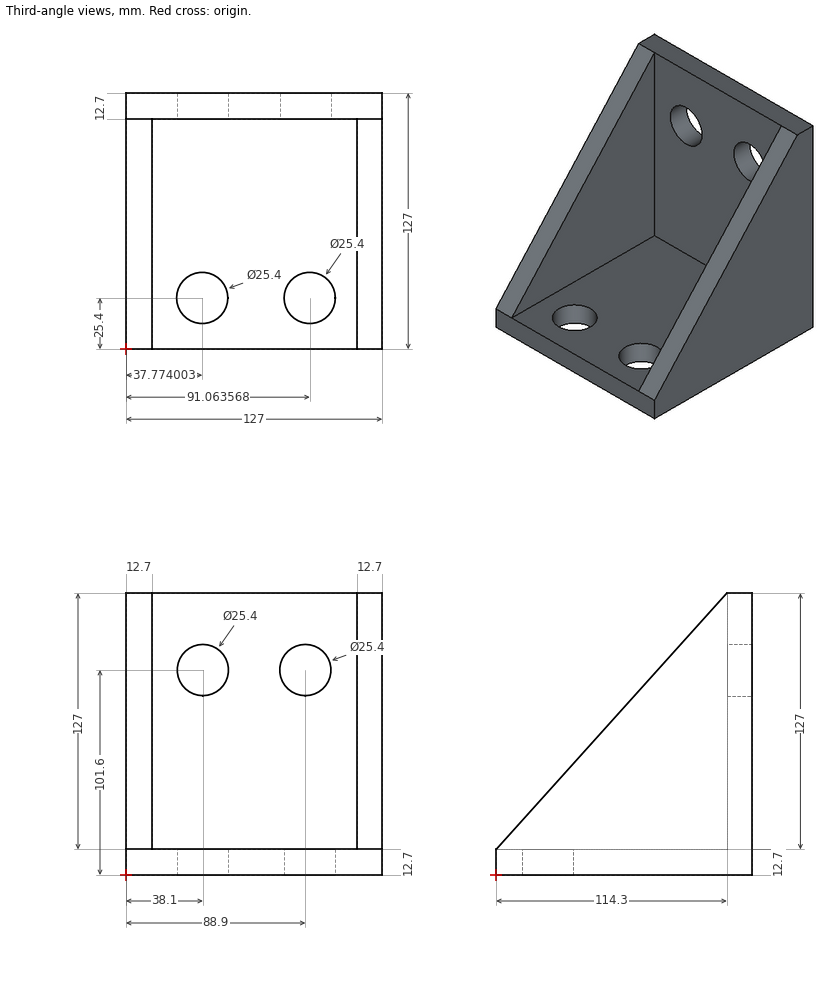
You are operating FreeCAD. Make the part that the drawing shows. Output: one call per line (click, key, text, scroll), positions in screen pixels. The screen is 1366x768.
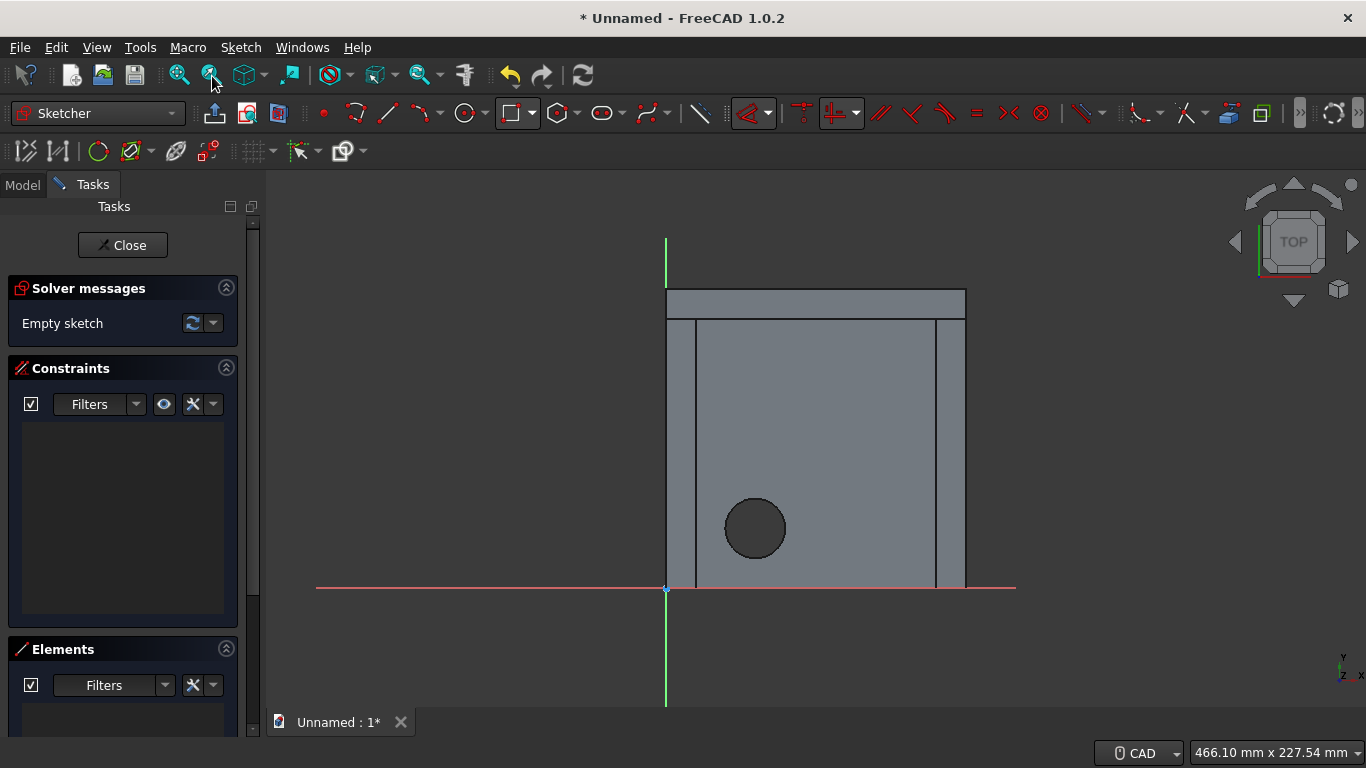
scroll(907, 546, up, 9)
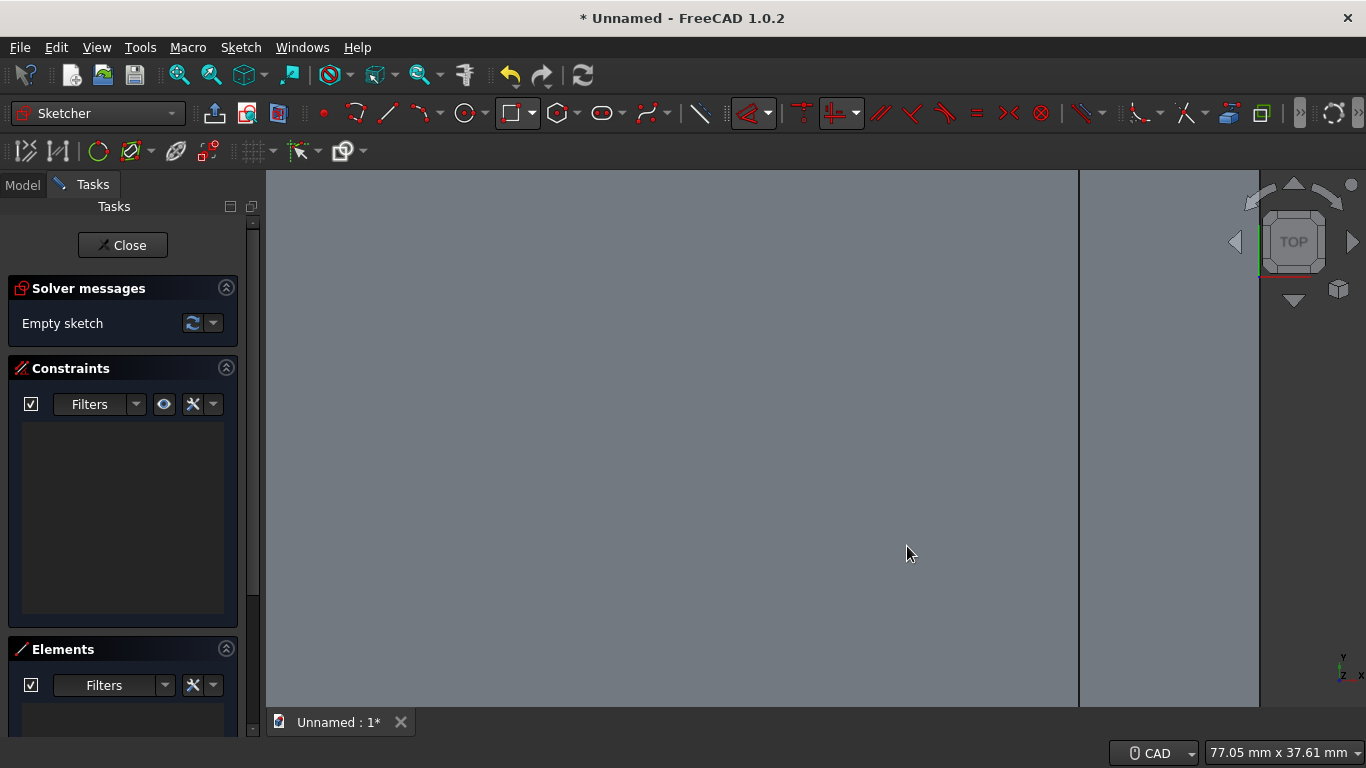
key(g)
key(c)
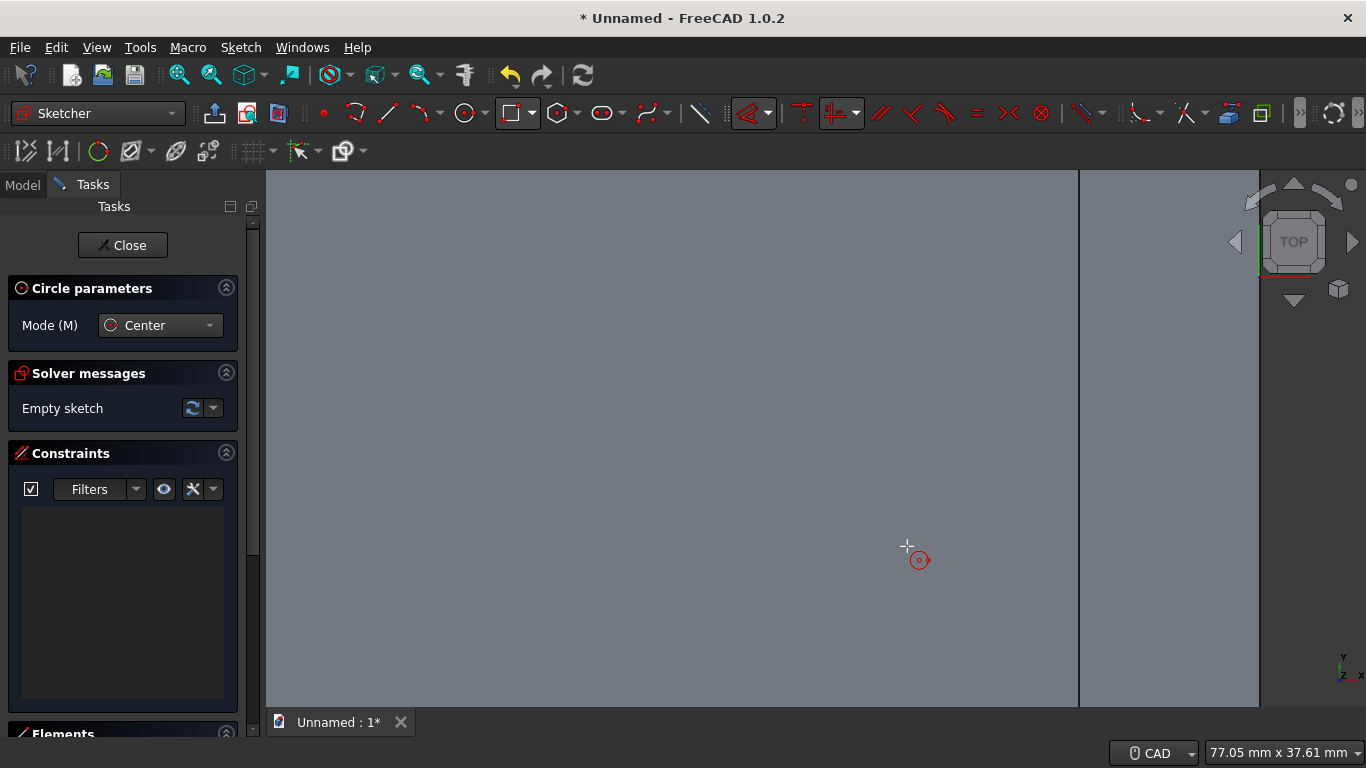
click(747, 436)
click(875, 308)
key(Escape)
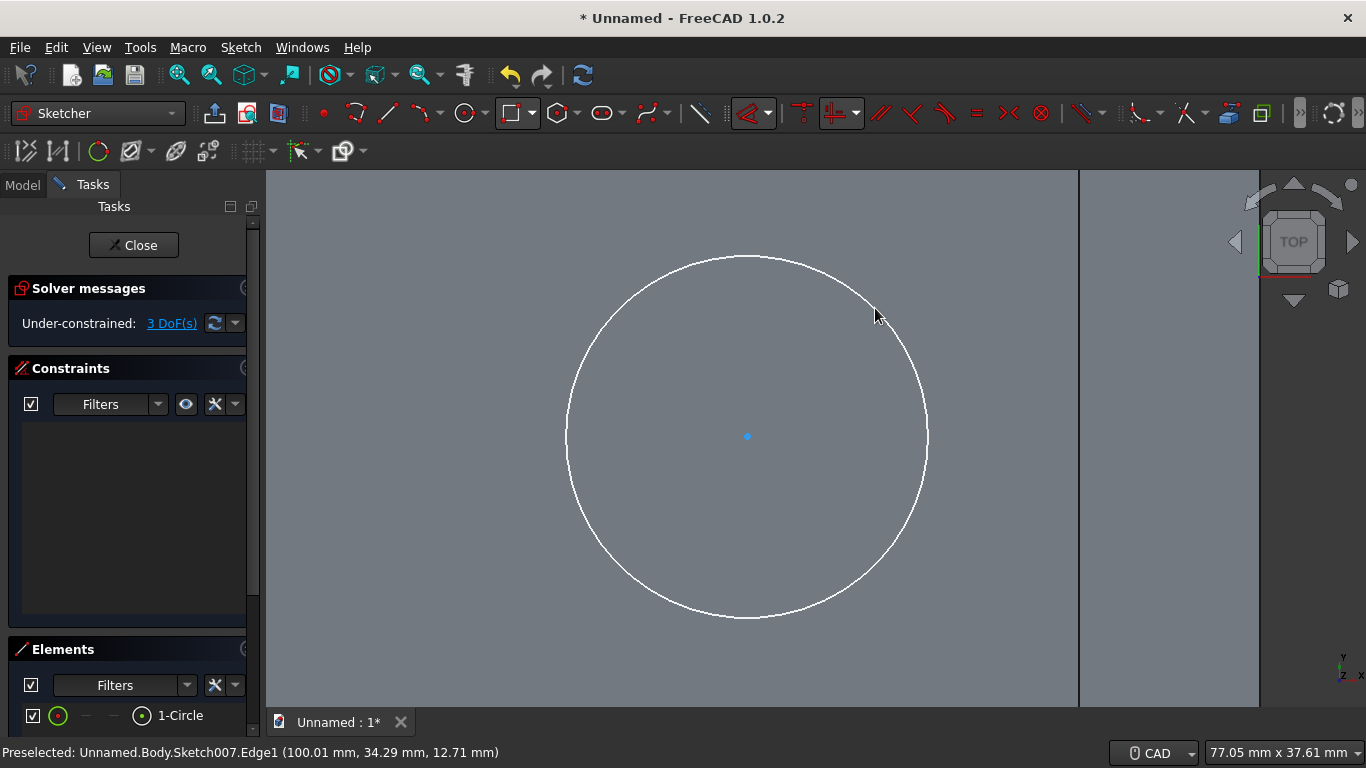
click(875, 309)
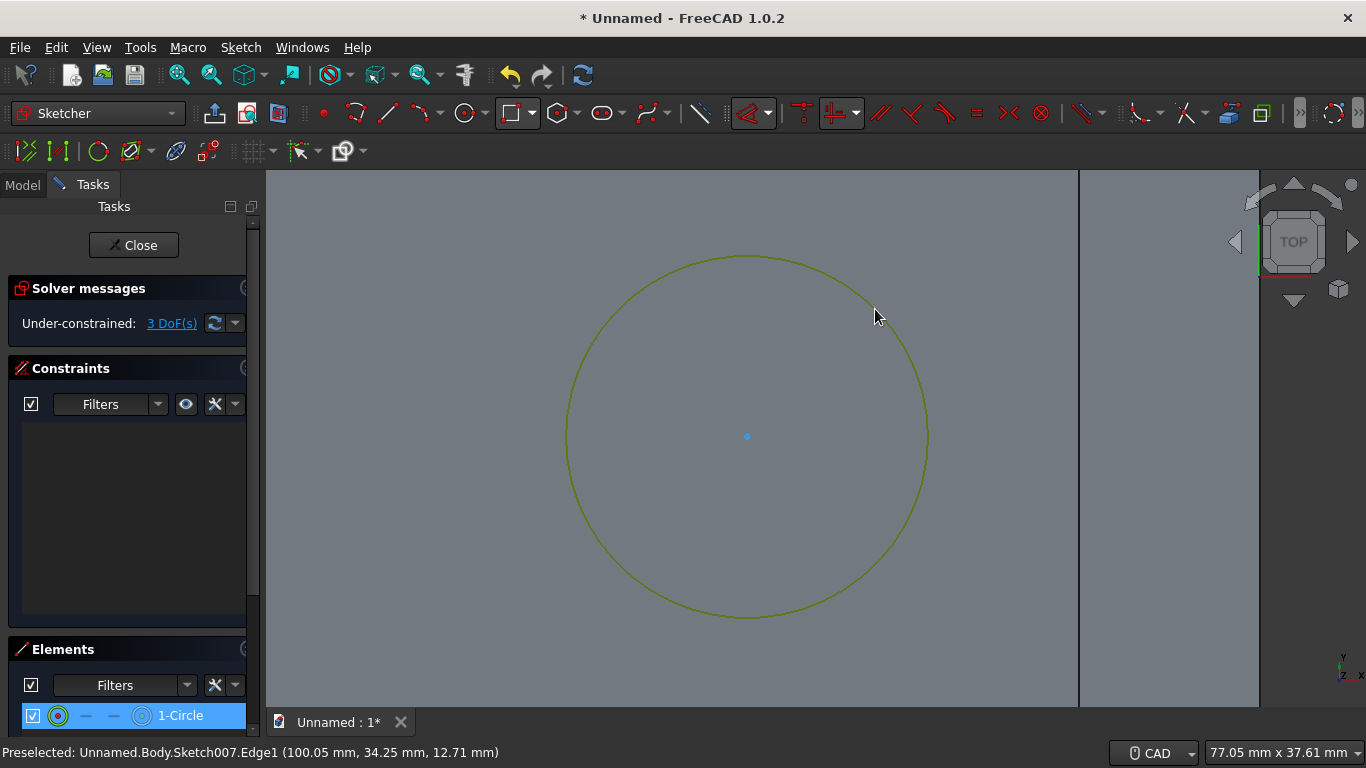
key(k)
key(o)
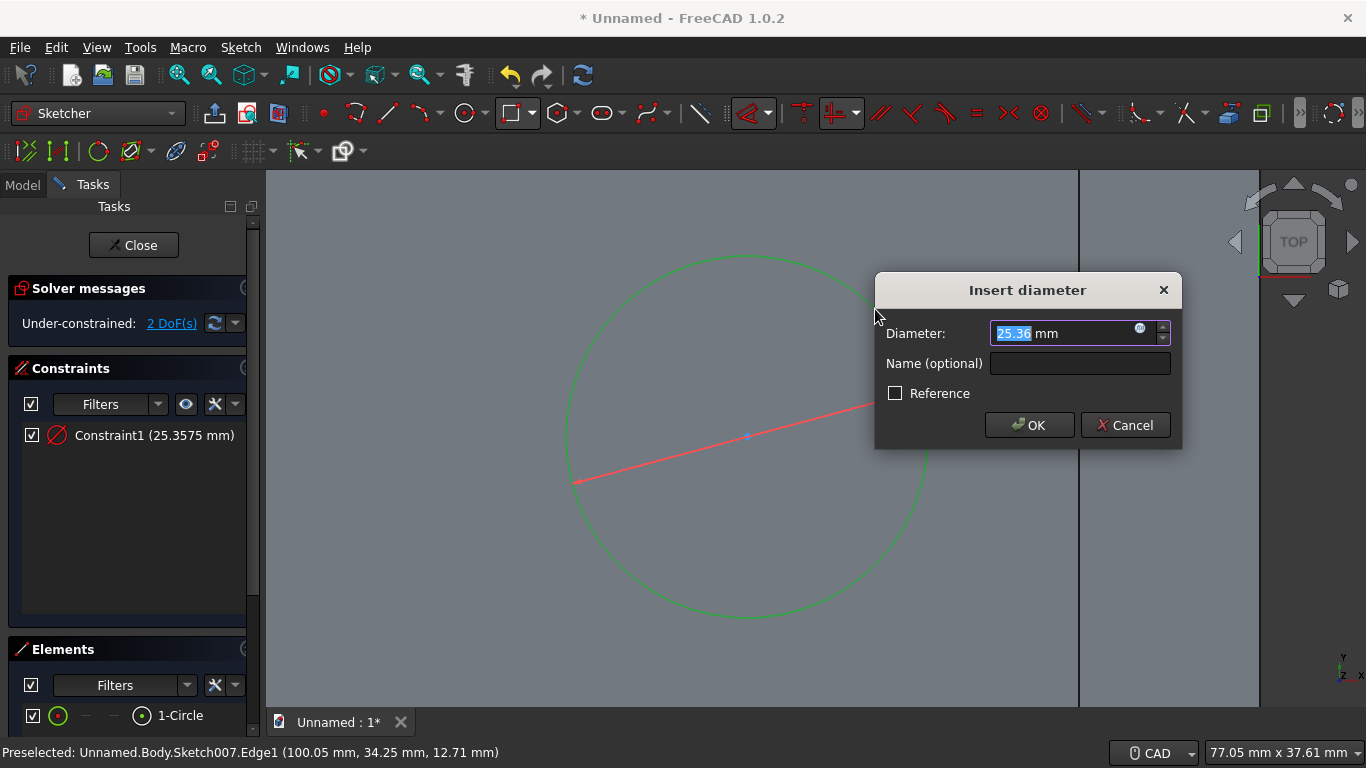
text(25.4)
key(Return)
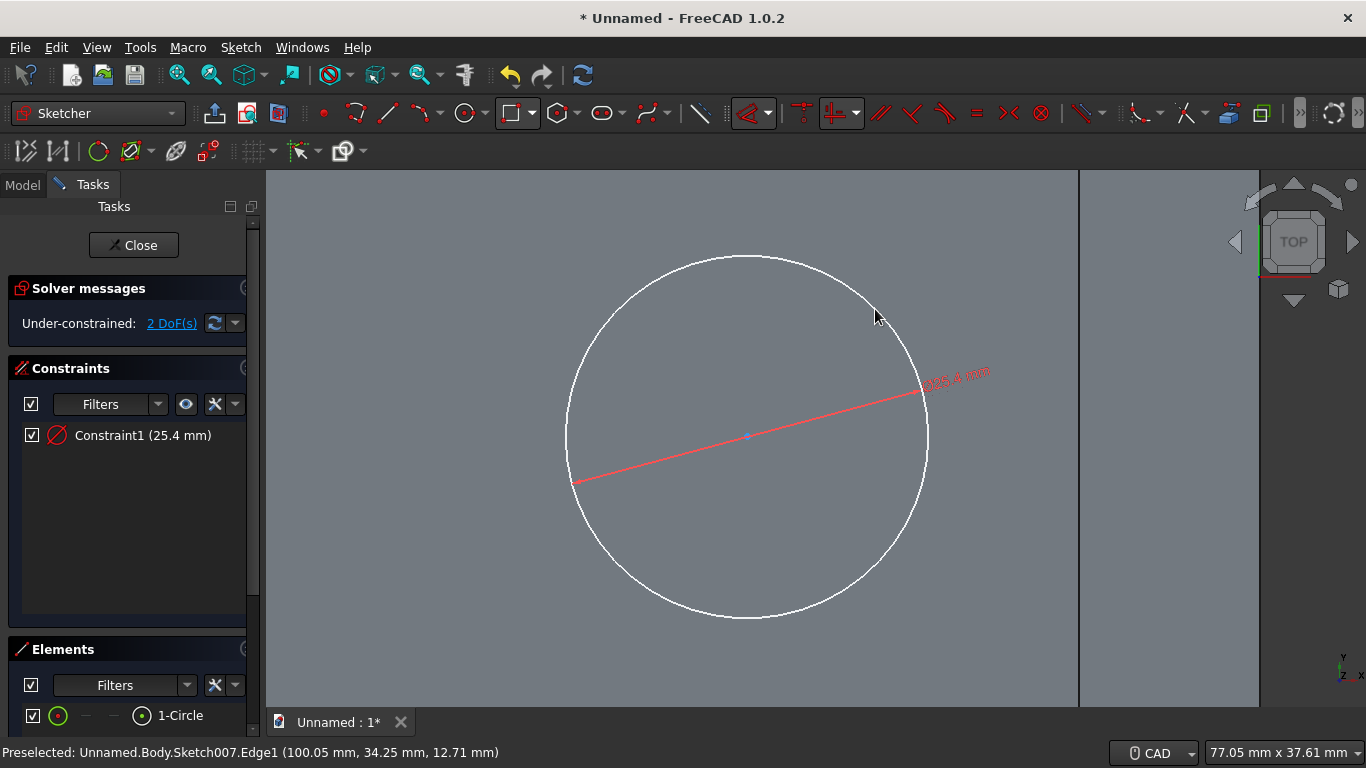
click(747, 437)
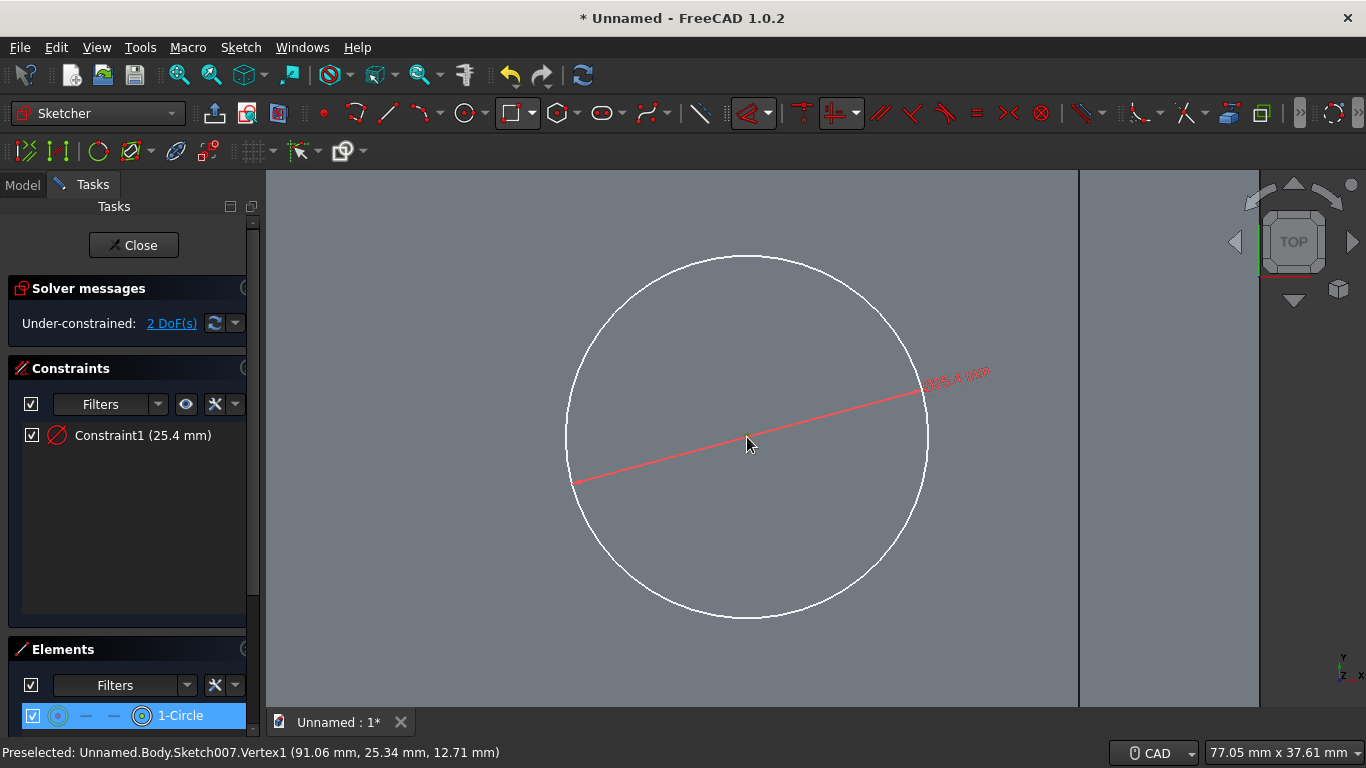
key(i)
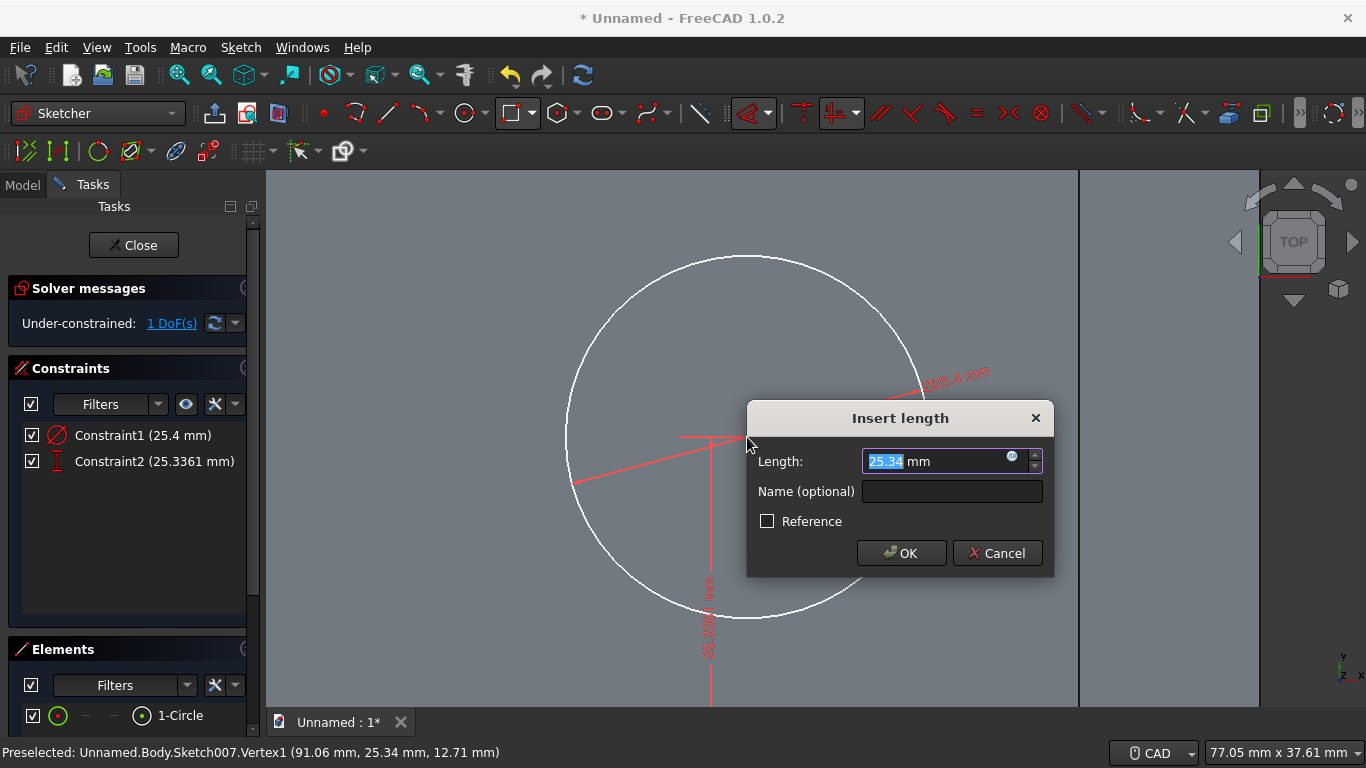
text(25.4)
key(Return)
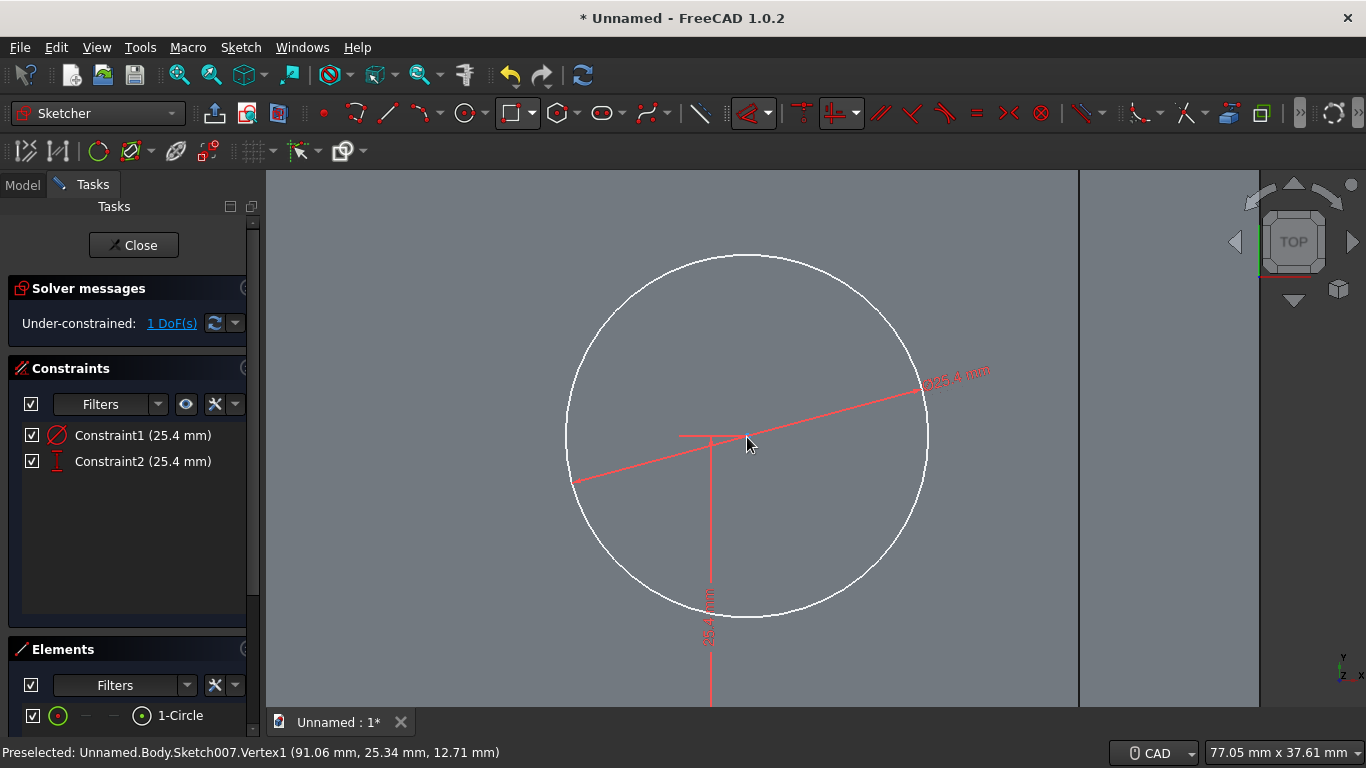
click(747, 436)